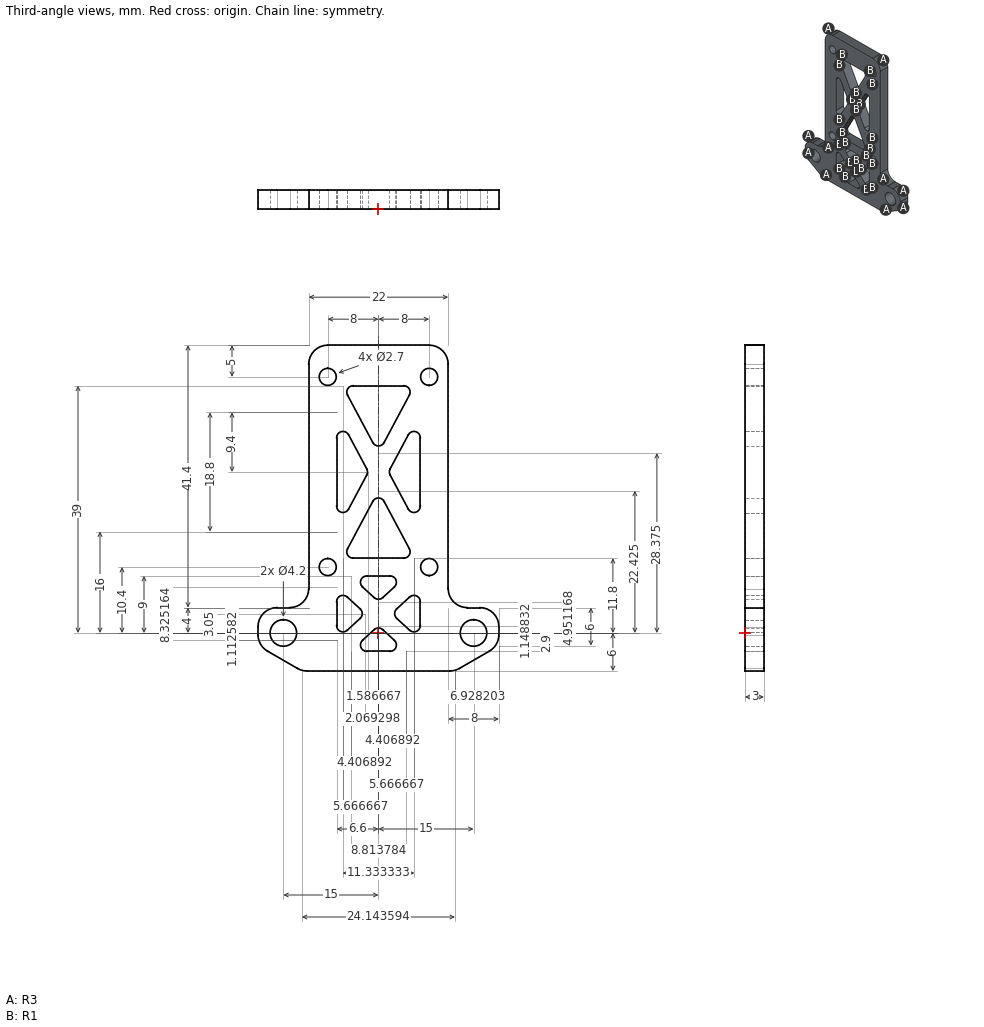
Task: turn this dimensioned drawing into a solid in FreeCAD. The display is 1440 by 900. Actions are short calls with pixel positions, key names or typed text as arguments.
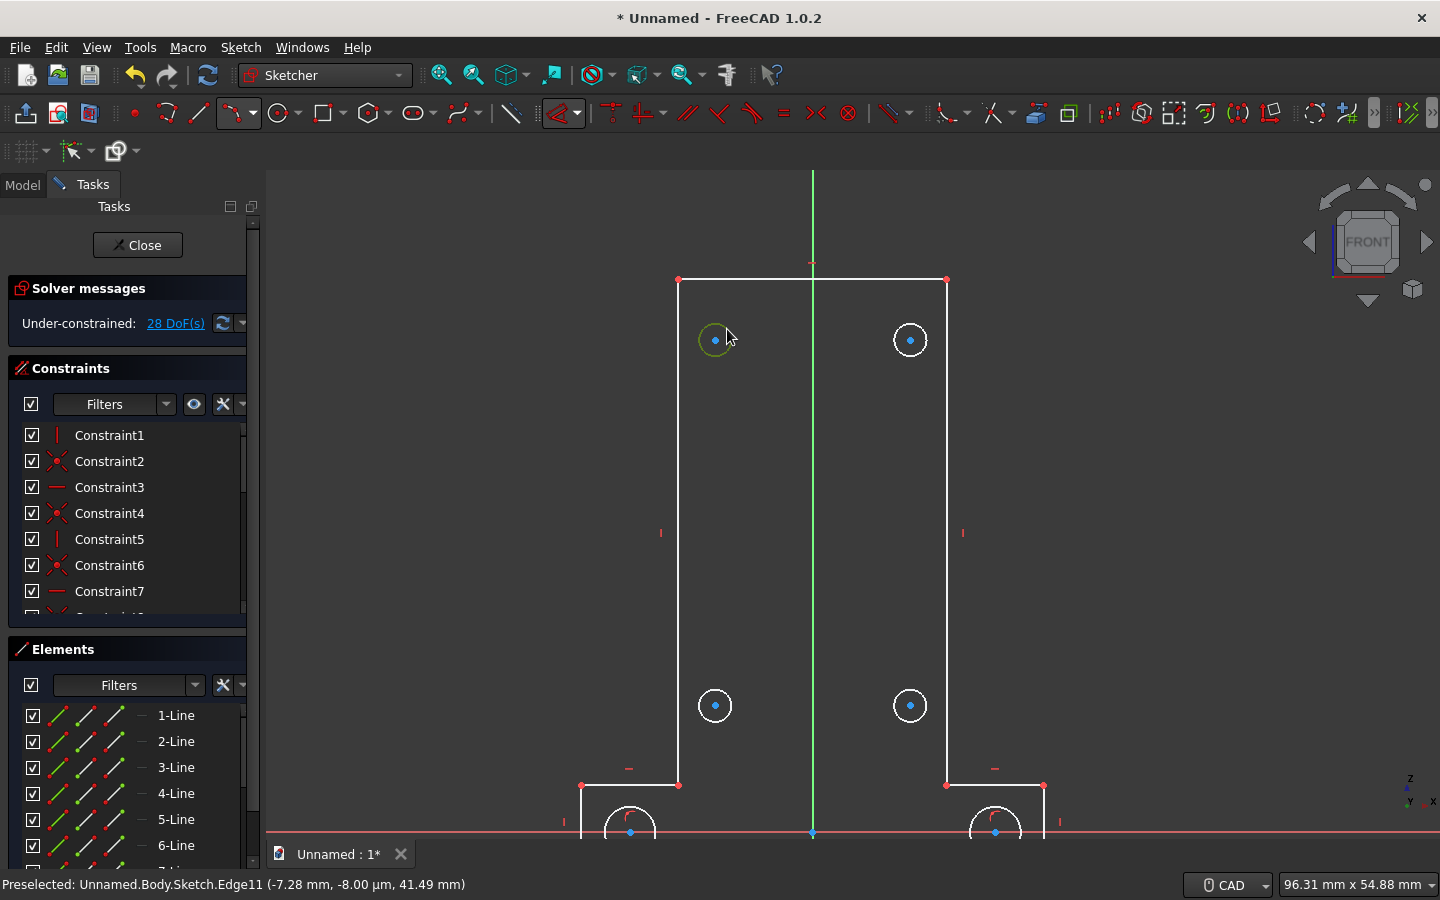
click(922, 329)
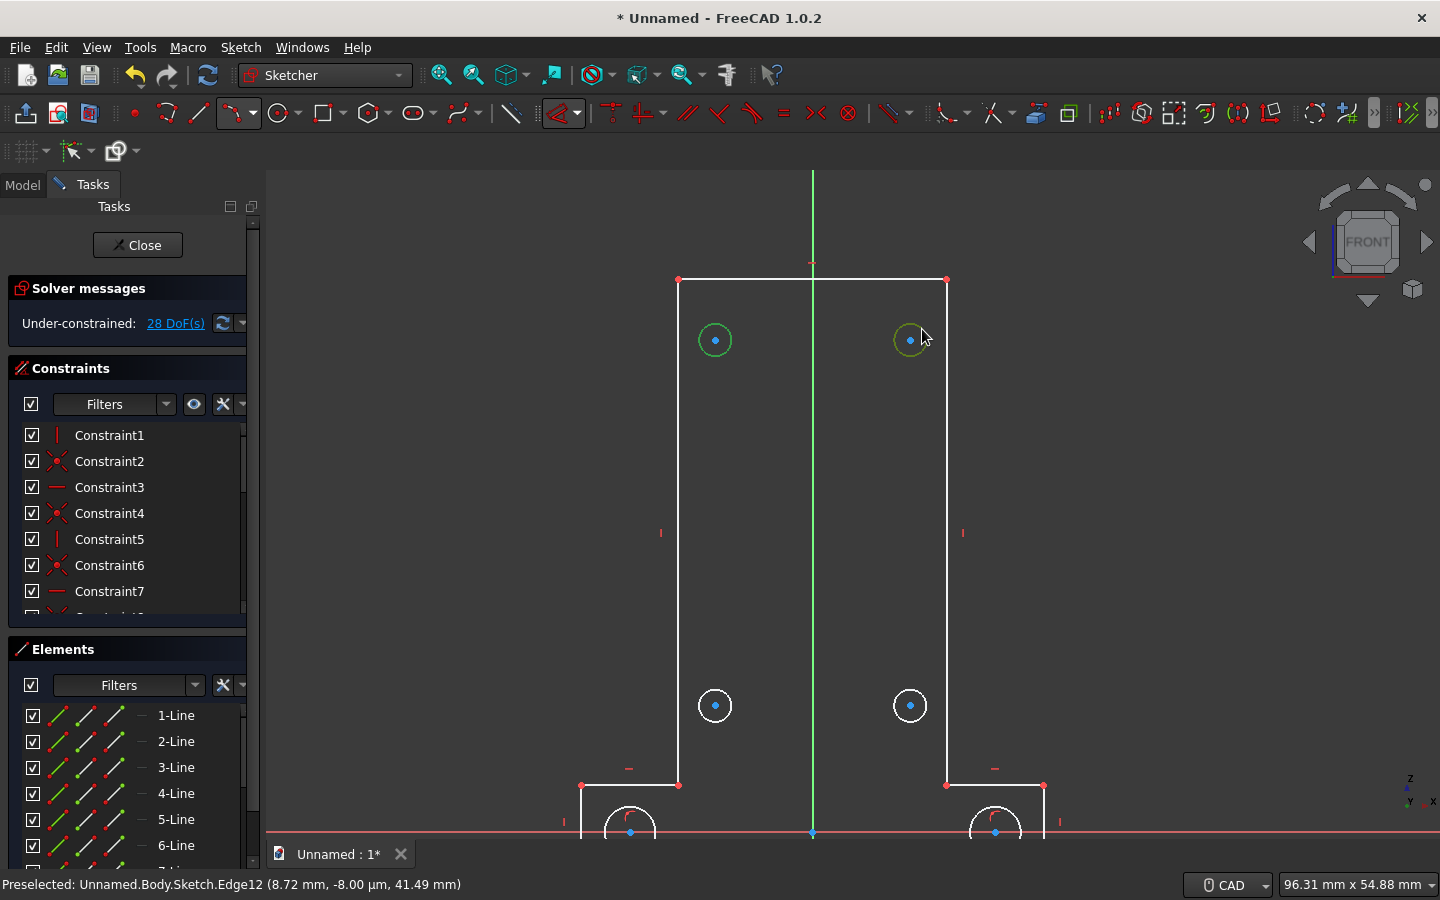
click(727, 694)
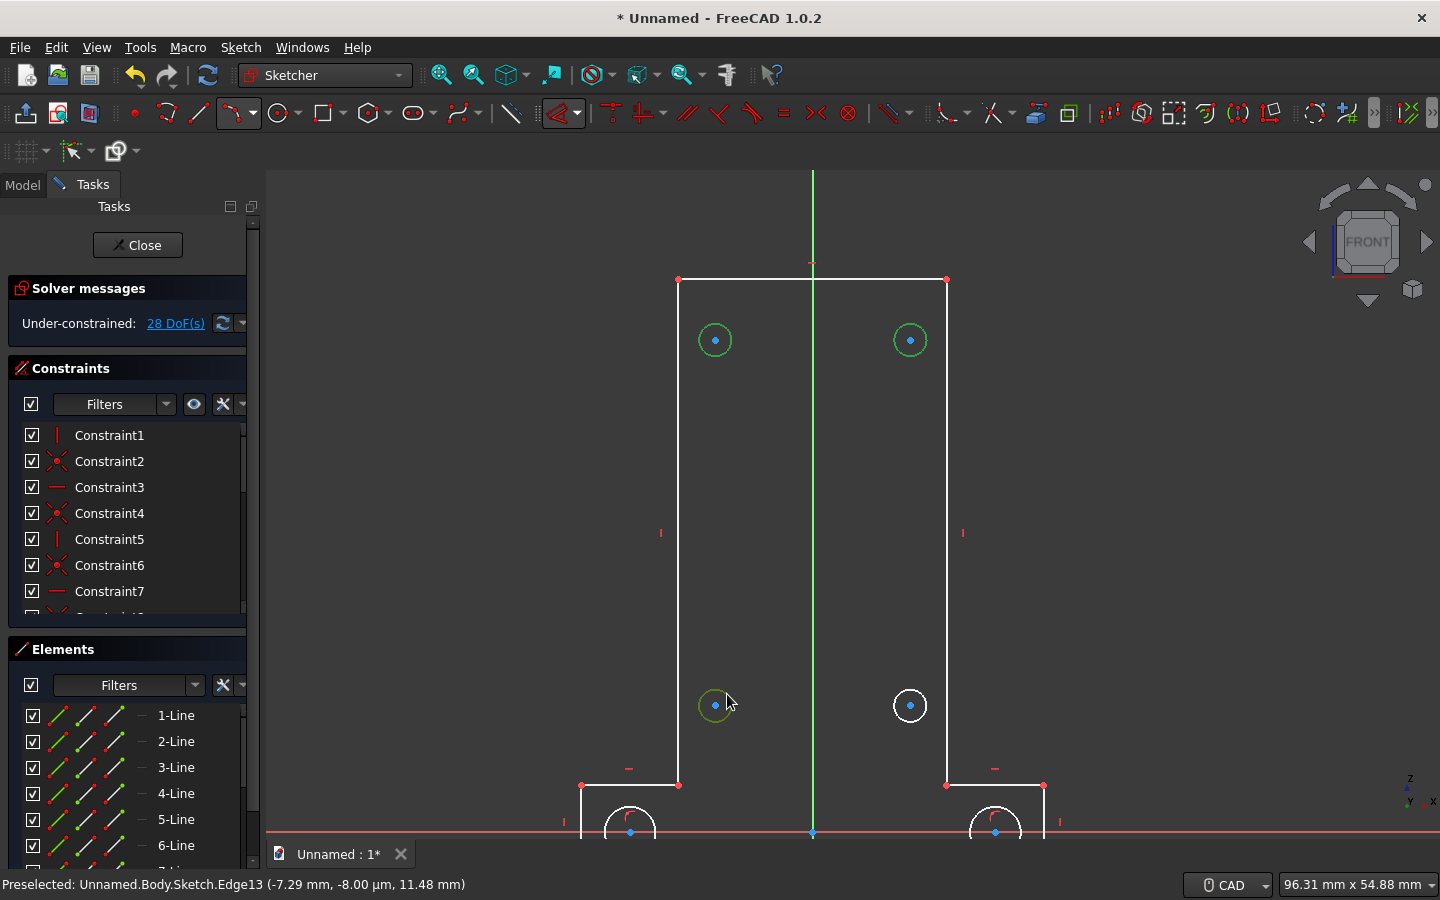
click(922, 694)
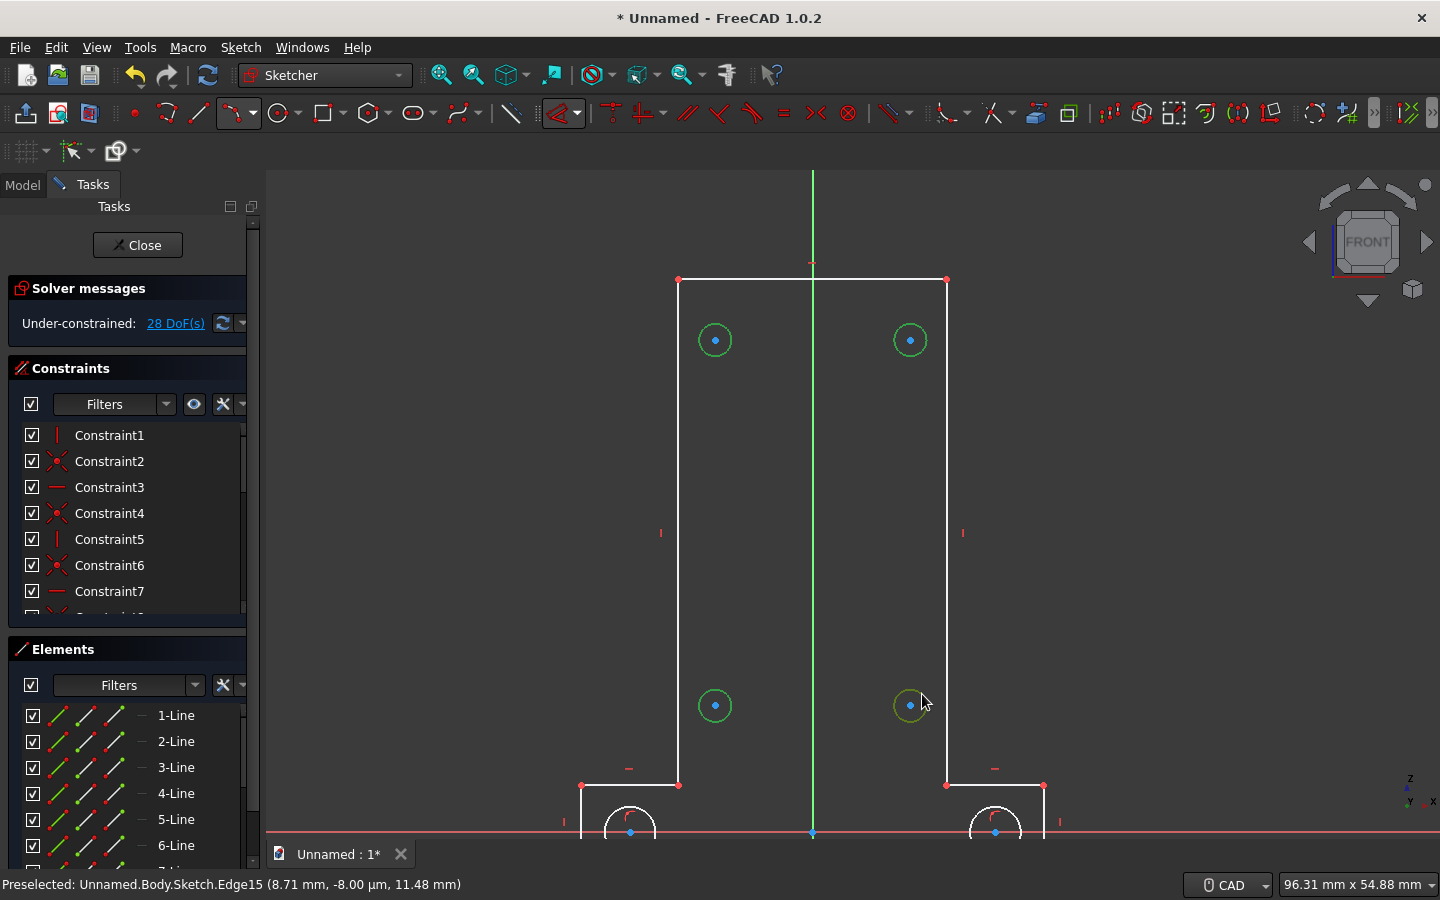
key(e)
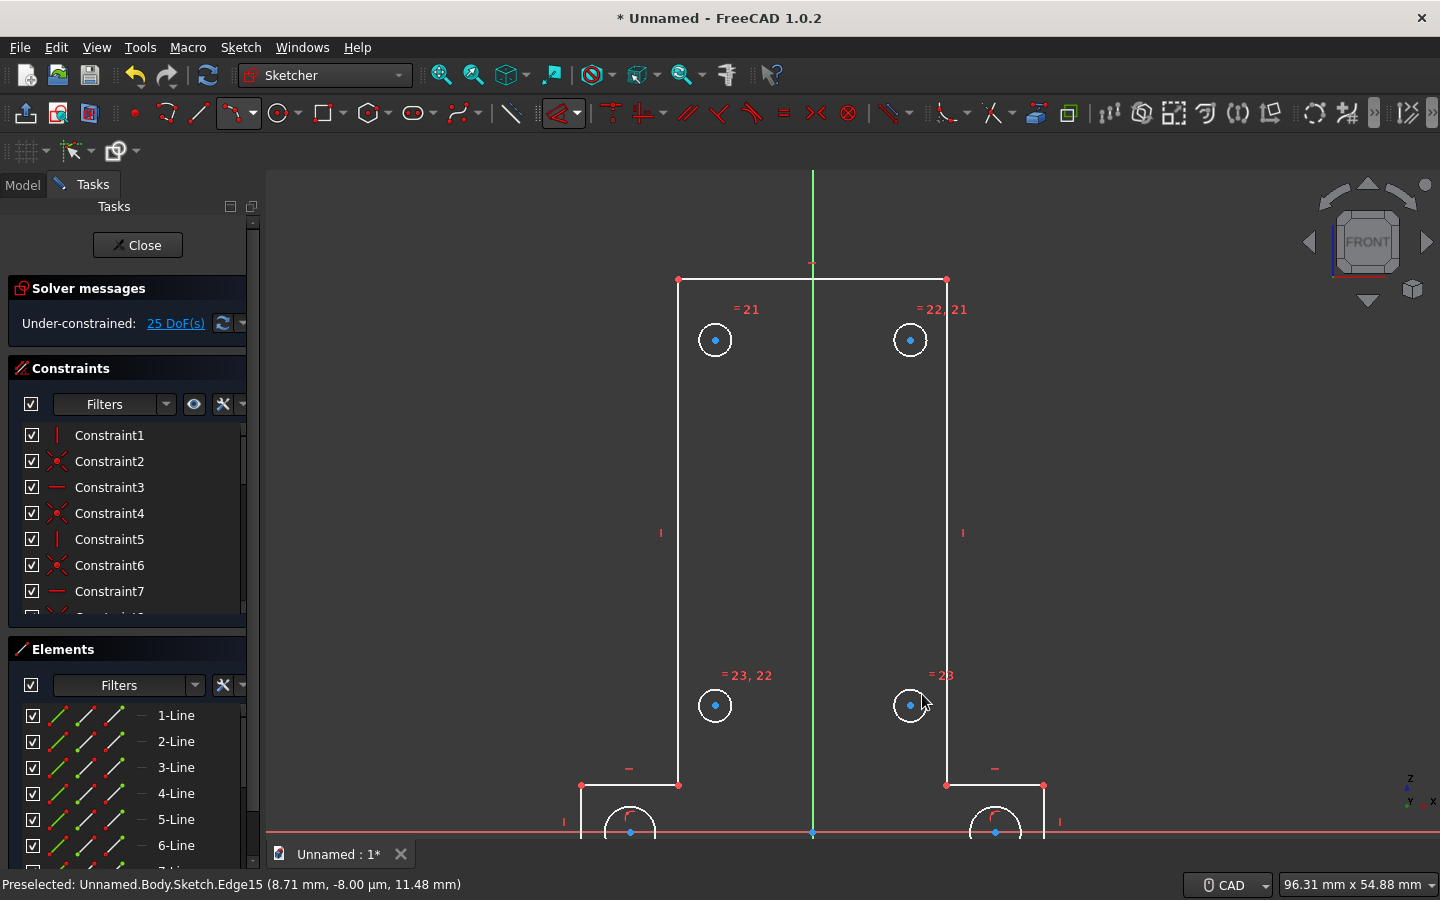
click(631, 807)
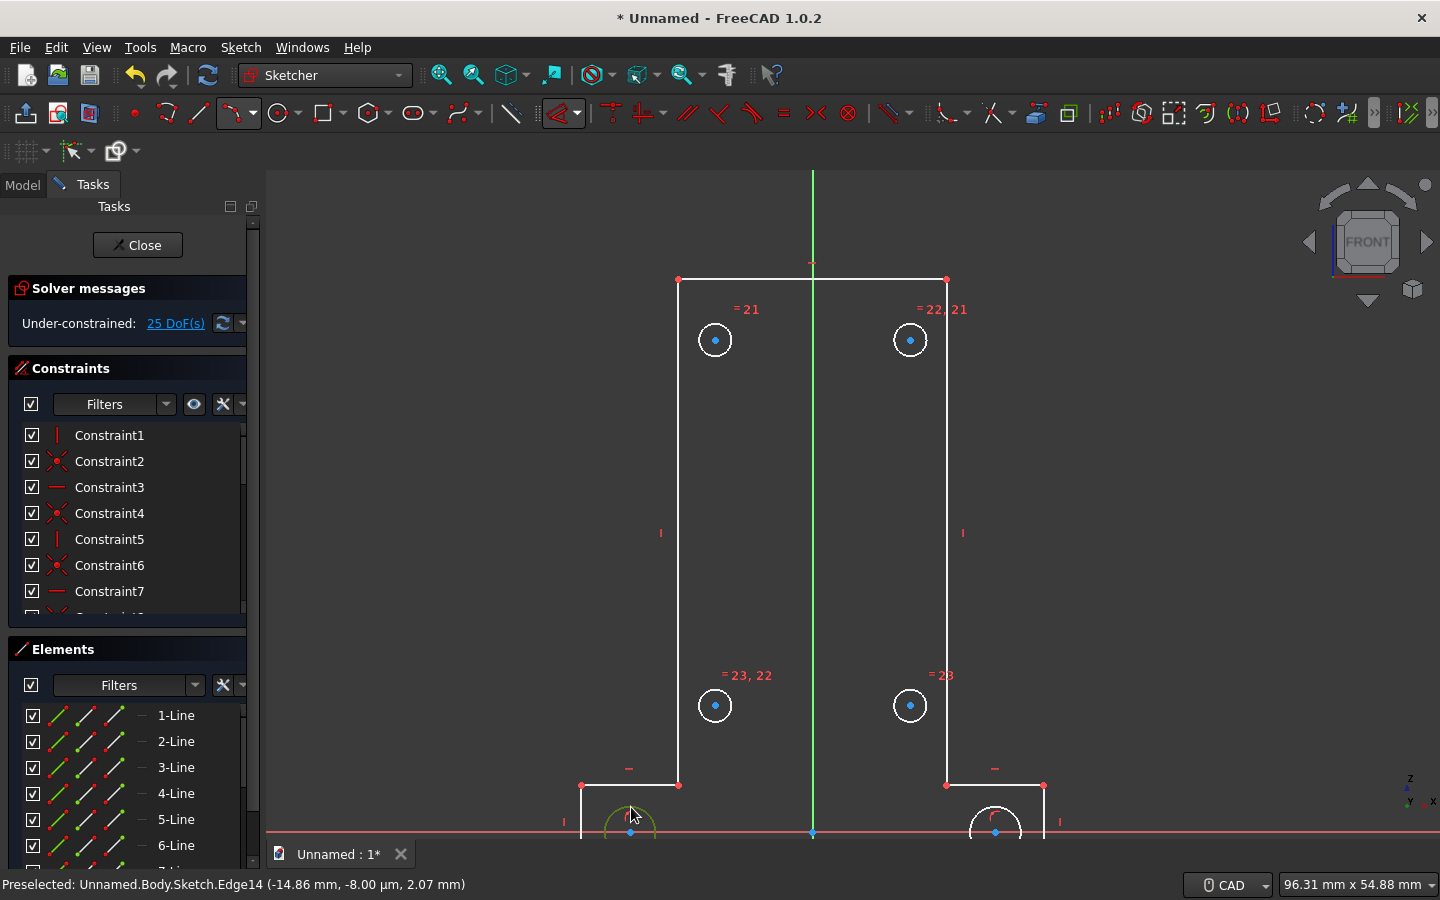
click(996, 807)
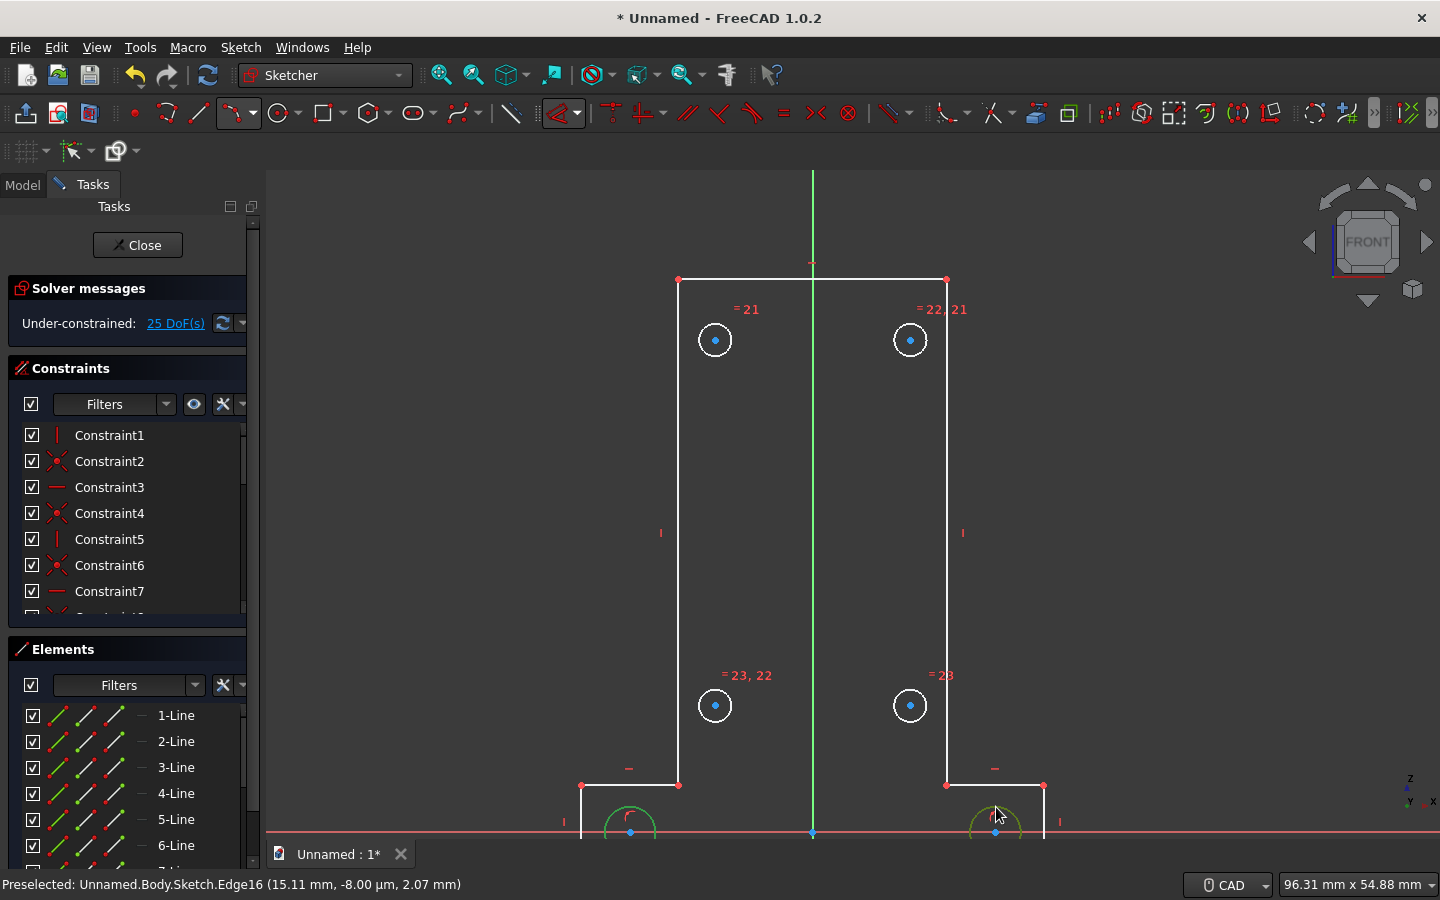
click(784, 114)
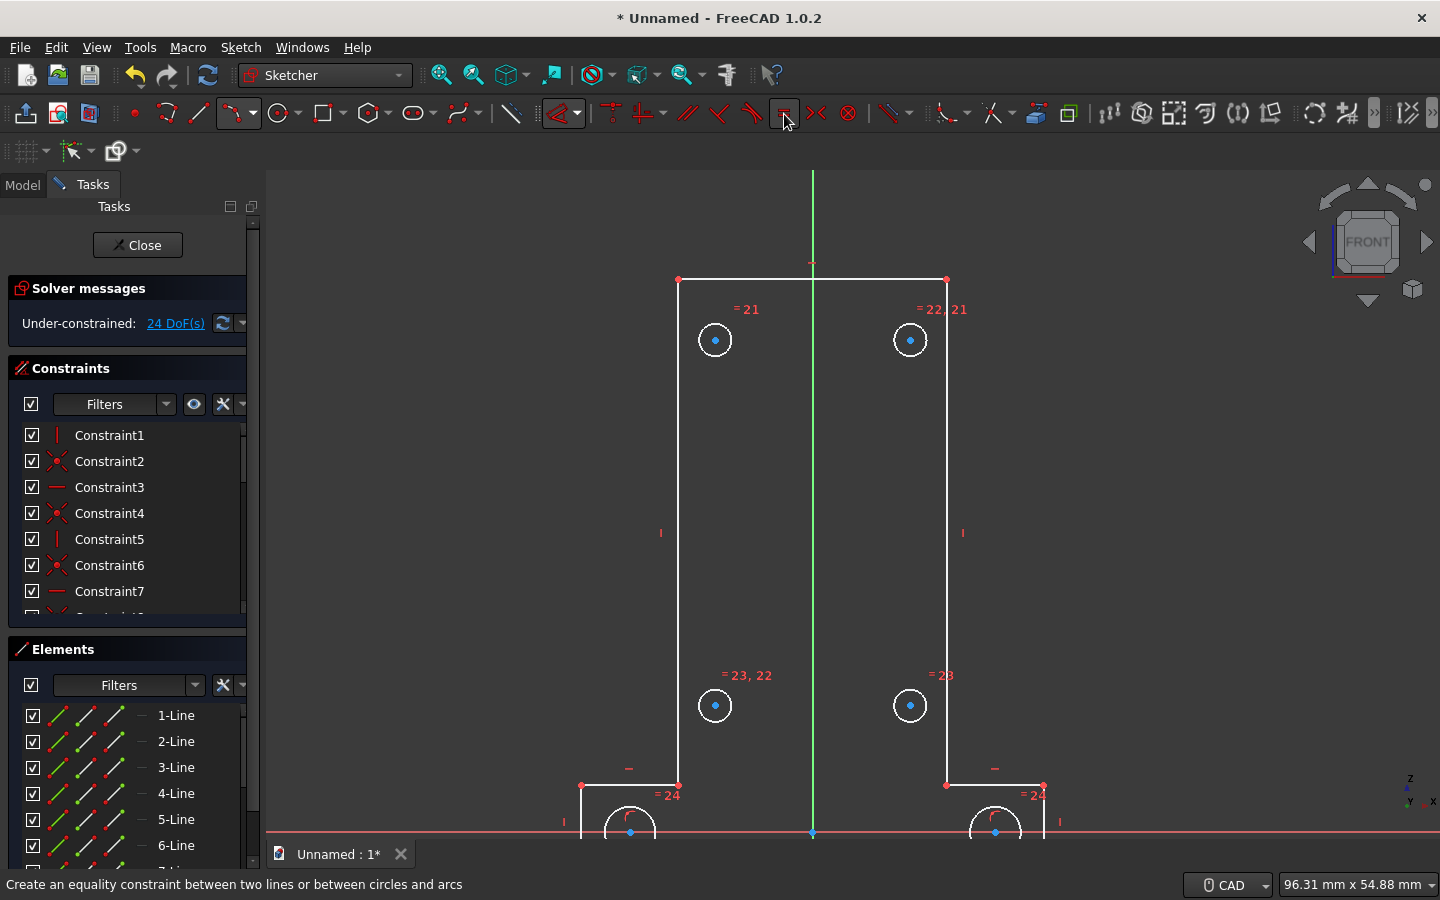
click(715, 340)